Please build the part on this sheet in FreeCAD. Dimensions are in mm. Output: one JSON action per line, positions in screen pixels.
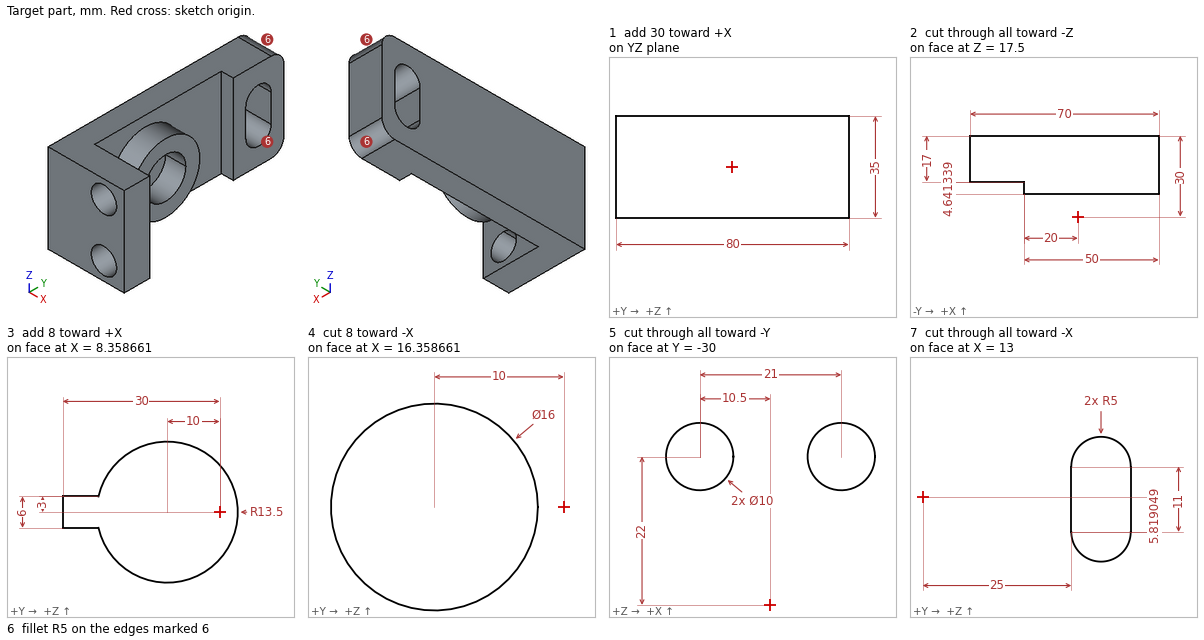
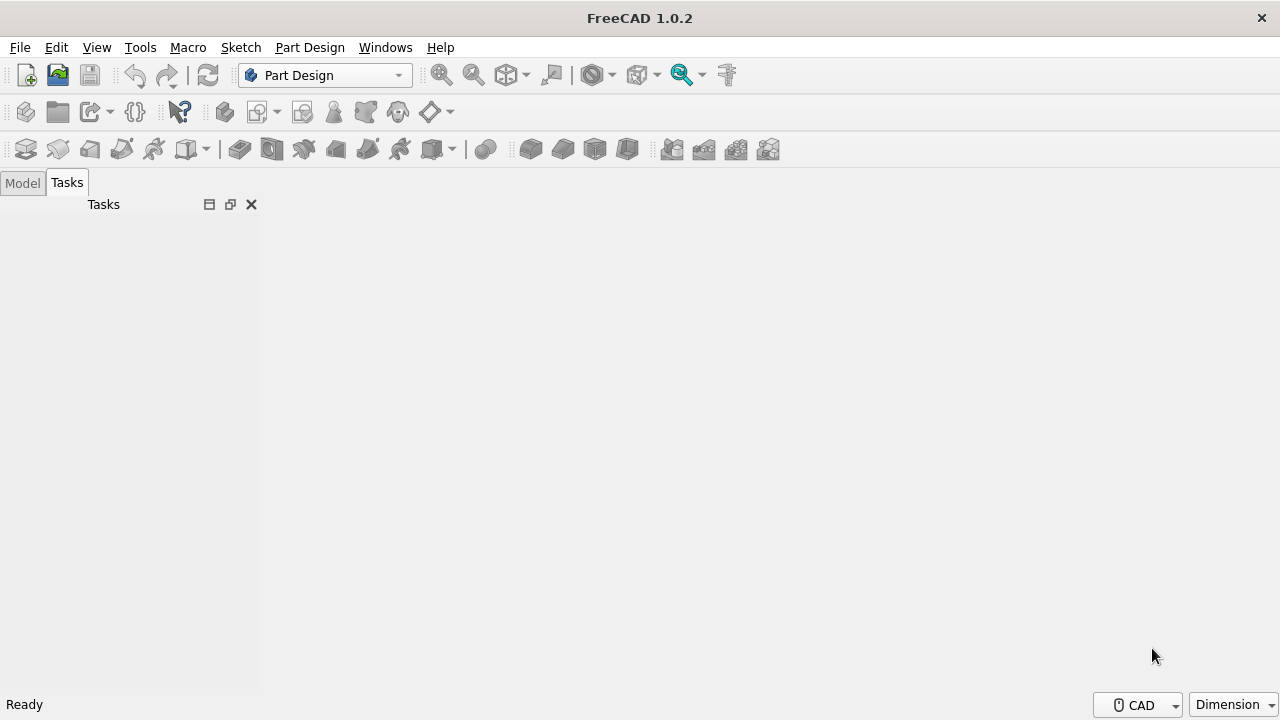
{"action": "left_click", "coordinate": [26, 76]}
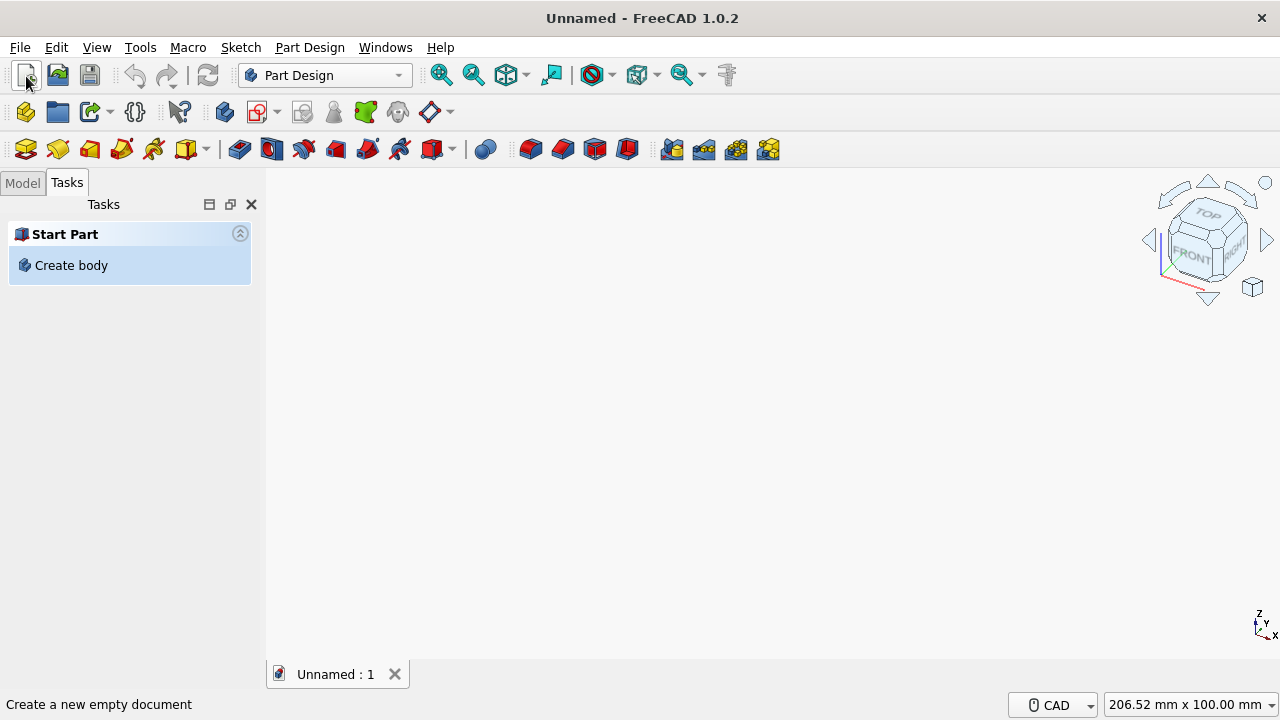
{"action": "left_click", "coordinate": [258, 112]}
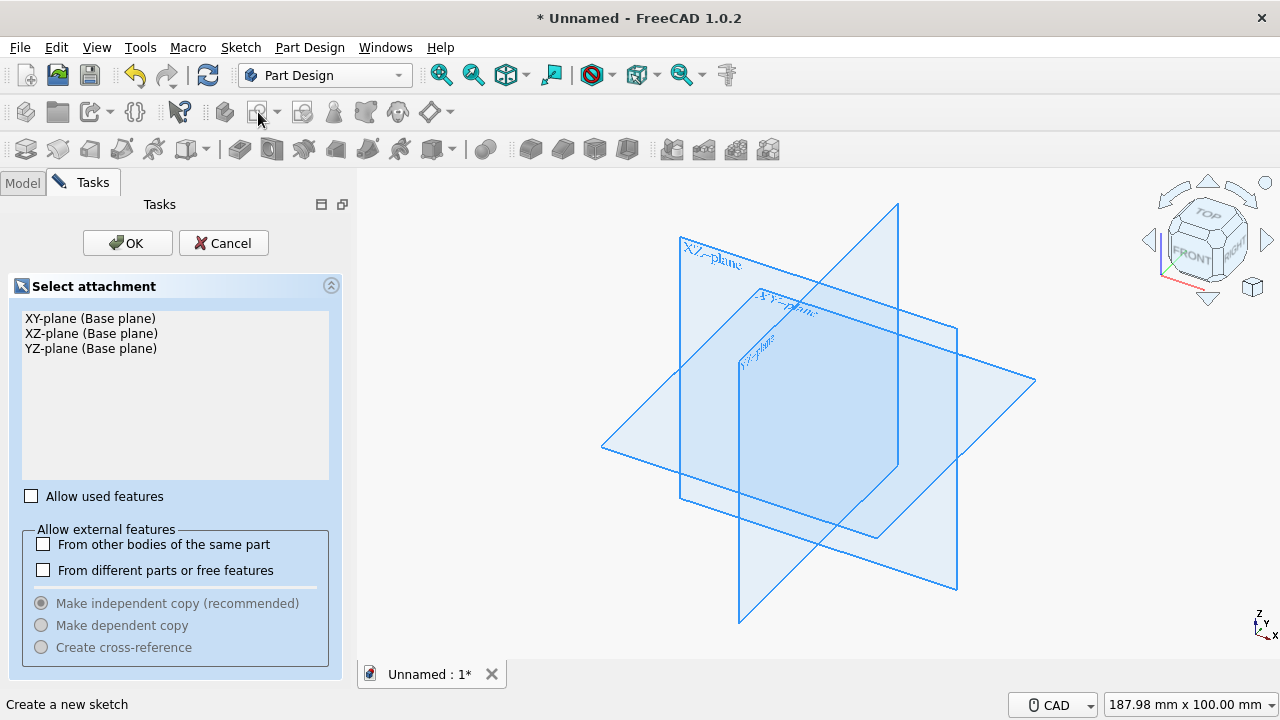
{"action": "left_click", "coordinate": [82, 348]}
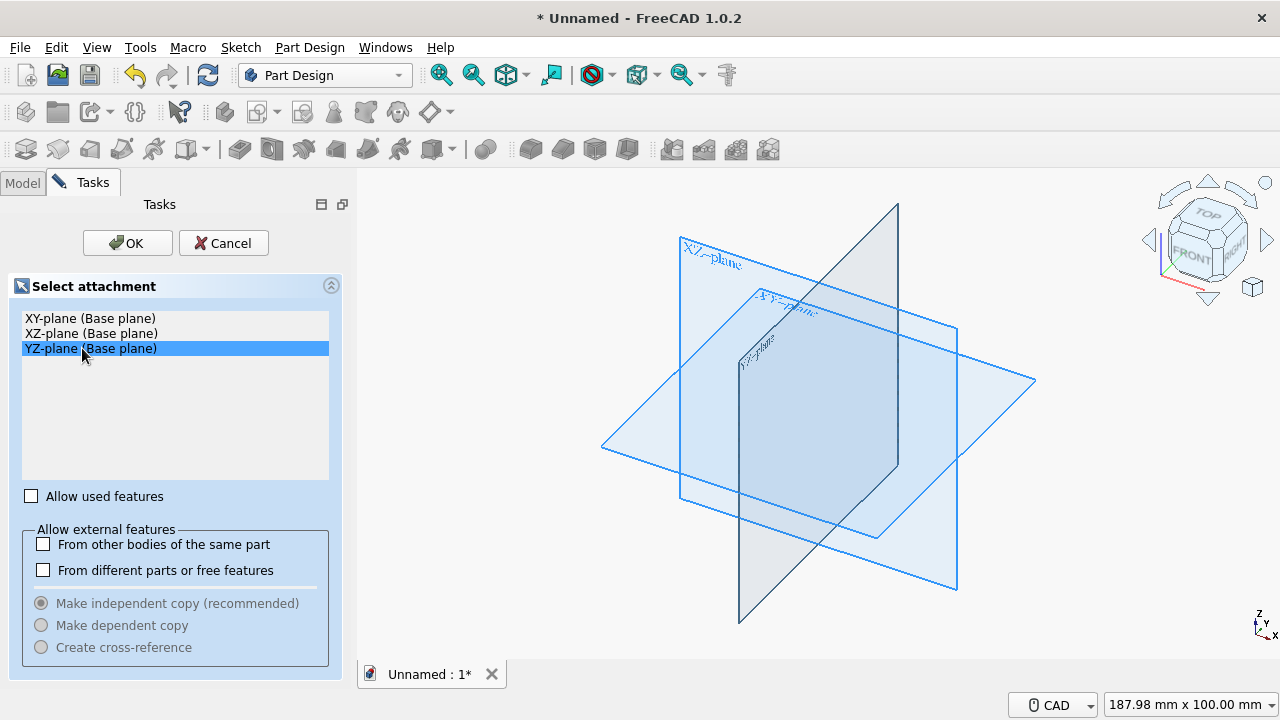
{"action": "left_click", "coordinate": [128, 243]}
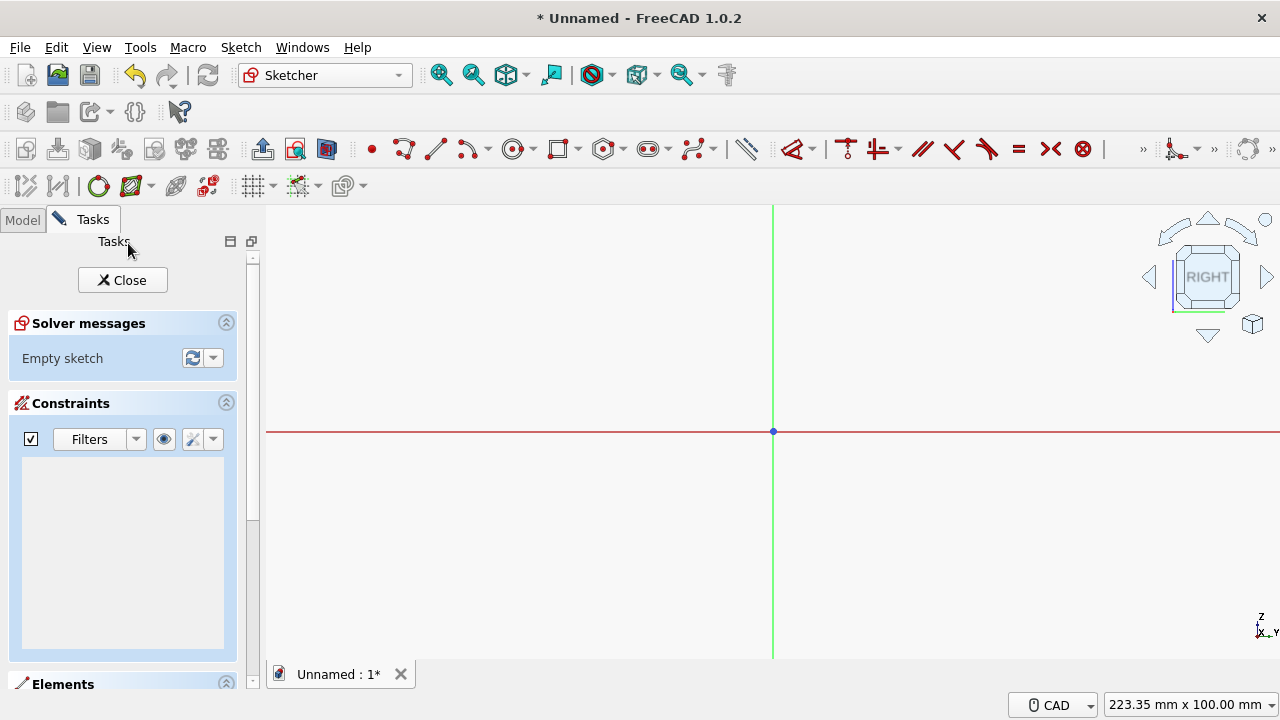
{"action": "scroll", "coordinate": [912, 432], "scroll_direction": "up", "scroll_amount": 2}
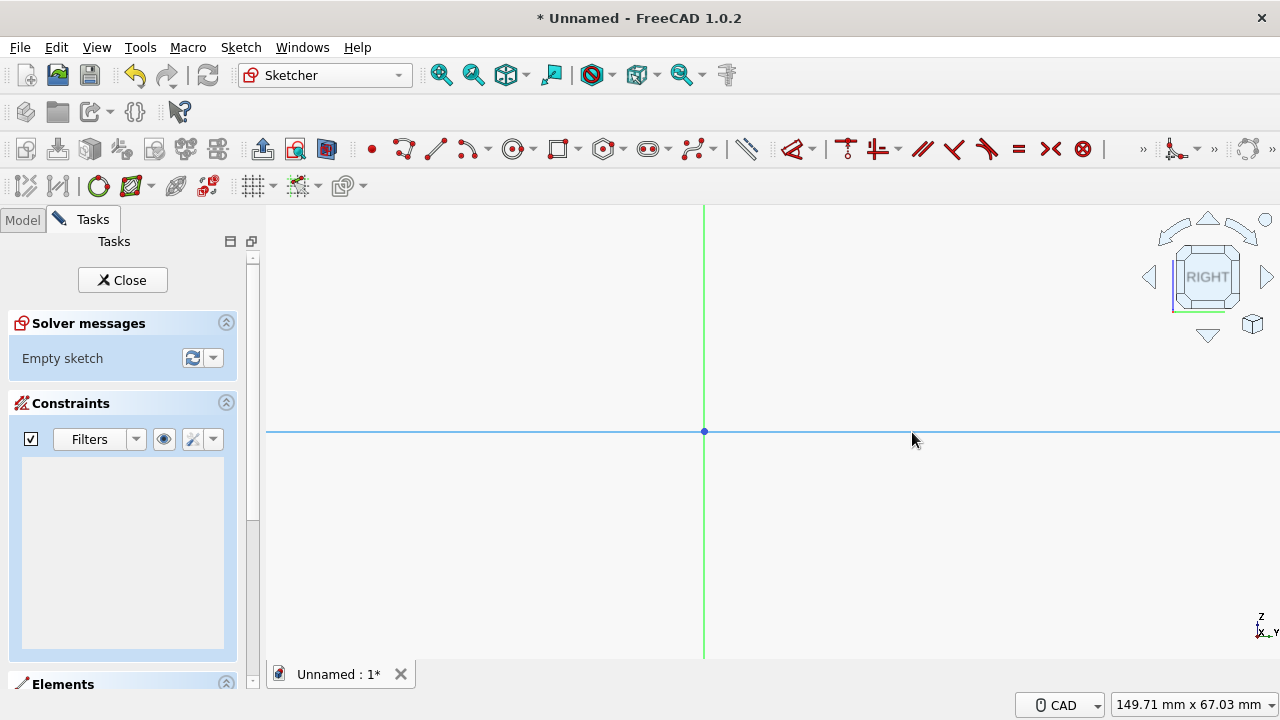
{"action": "key", "text": "g v"}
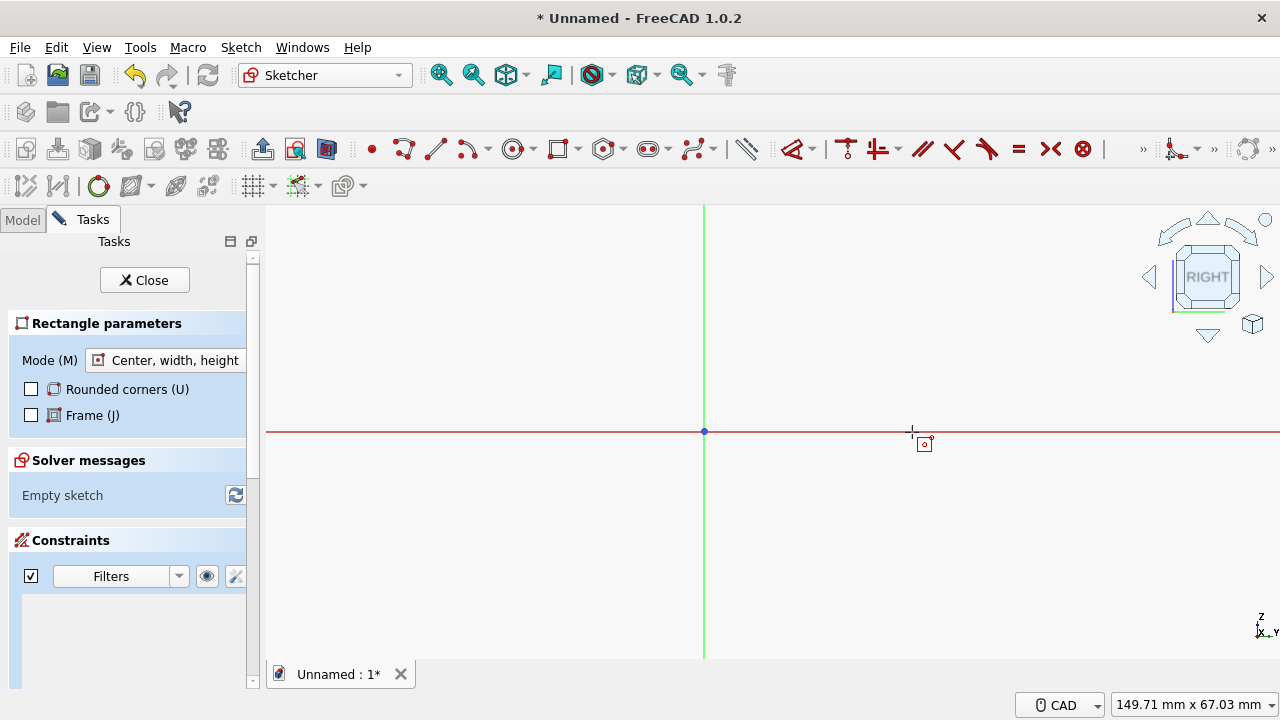
{"action": "left_click", "coordinate": [704, 432]}
{"action": "left_click", "coordinate": [975, 313]}
{"action": "key", "text": "Escape"}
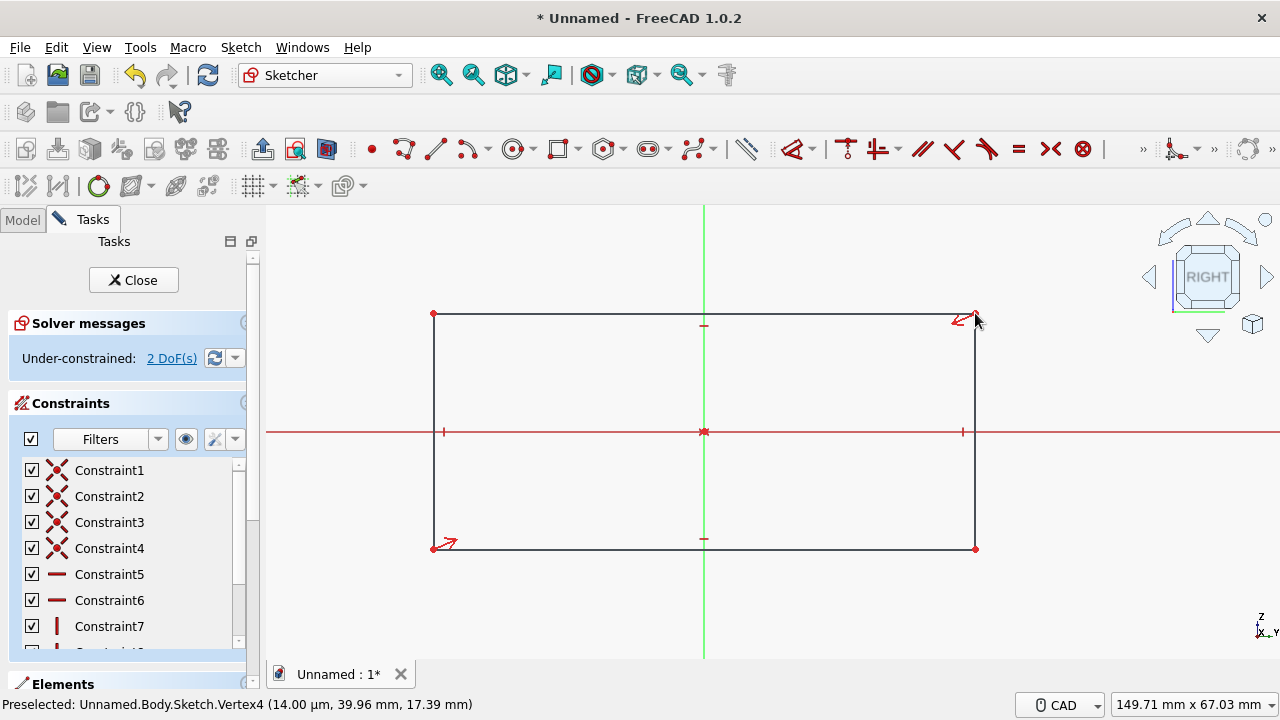
{"action": "left_click", "coordinate": [792, 150]}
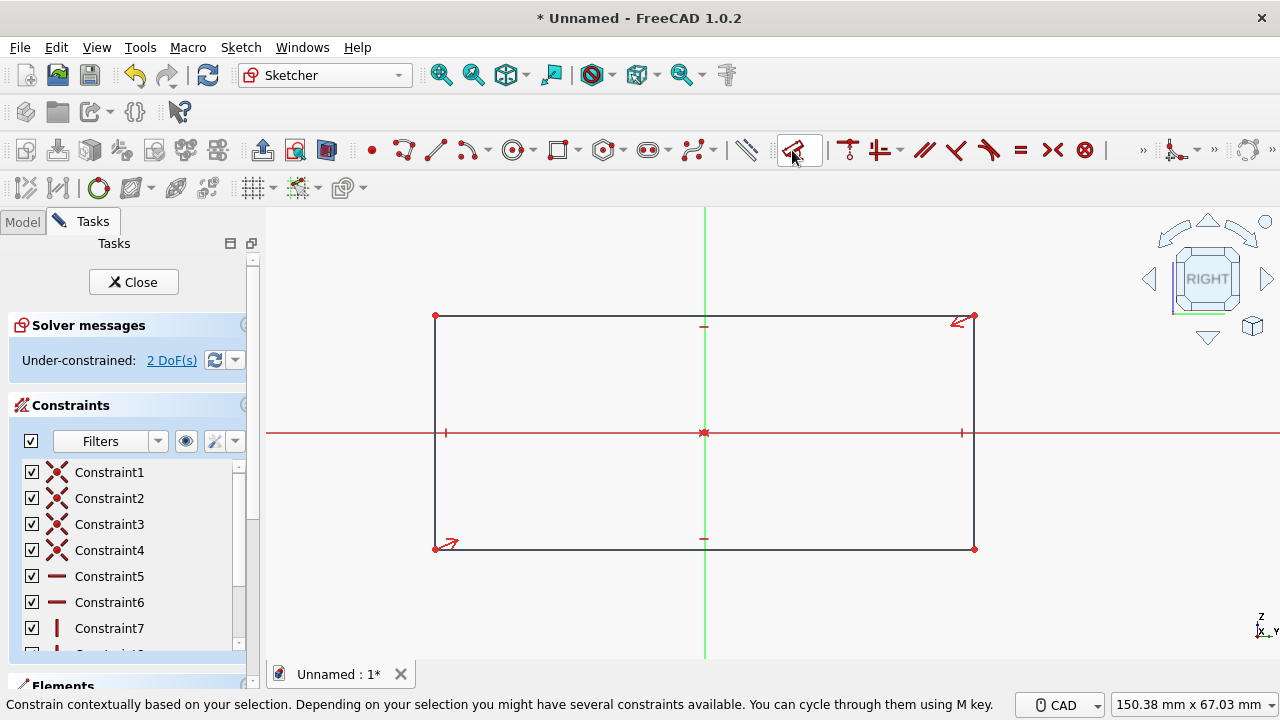
{"action": "left_click", "coordinate": [597, 550]}
{"action": "left_click", "coordinate": [581, 584]}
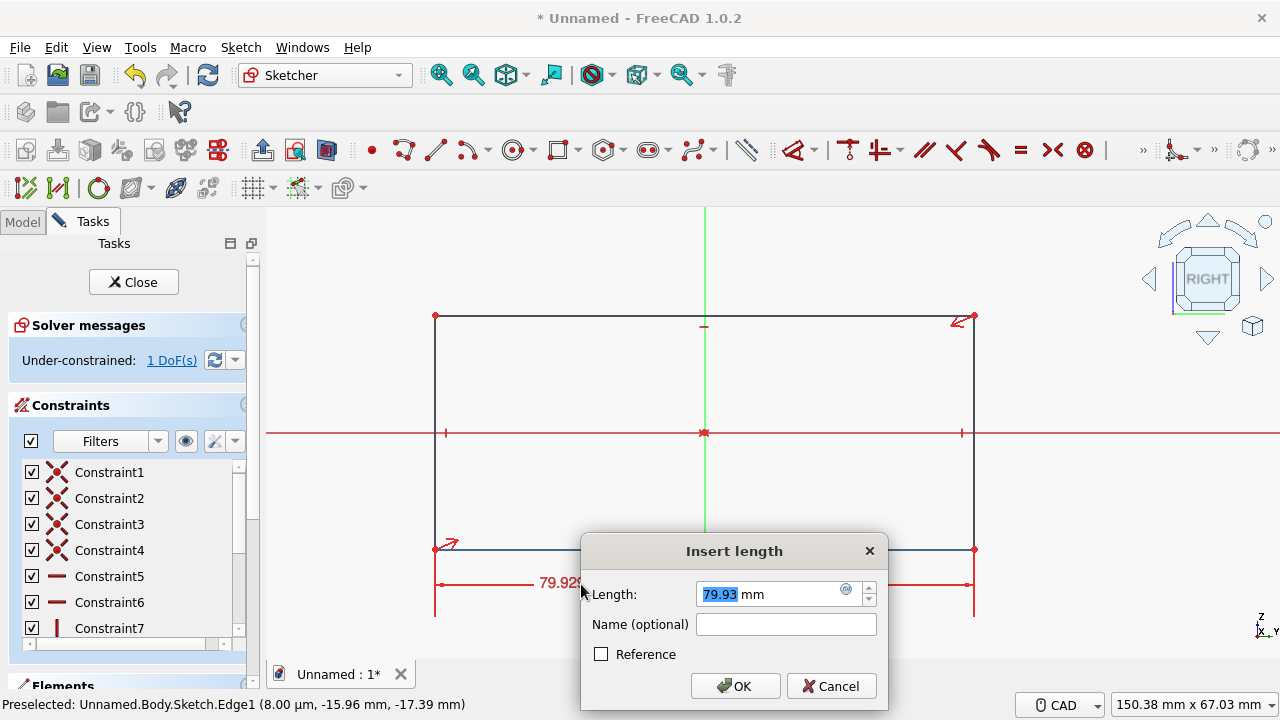
{"action": "type", "text": "80"}
{"action": "key", "text": "Return"}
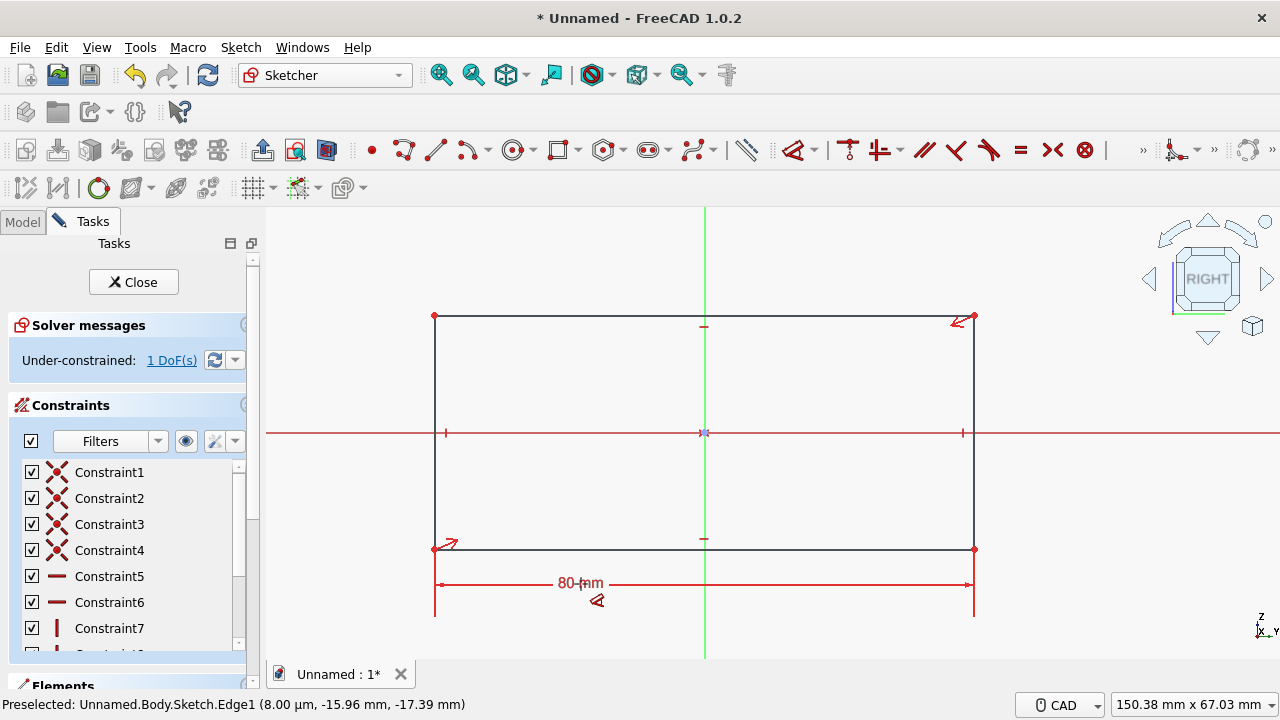
{"action": "left_click", "coordinate": [974, 480]}
{"action": "left_click", "coordinate": [1008, 379]}